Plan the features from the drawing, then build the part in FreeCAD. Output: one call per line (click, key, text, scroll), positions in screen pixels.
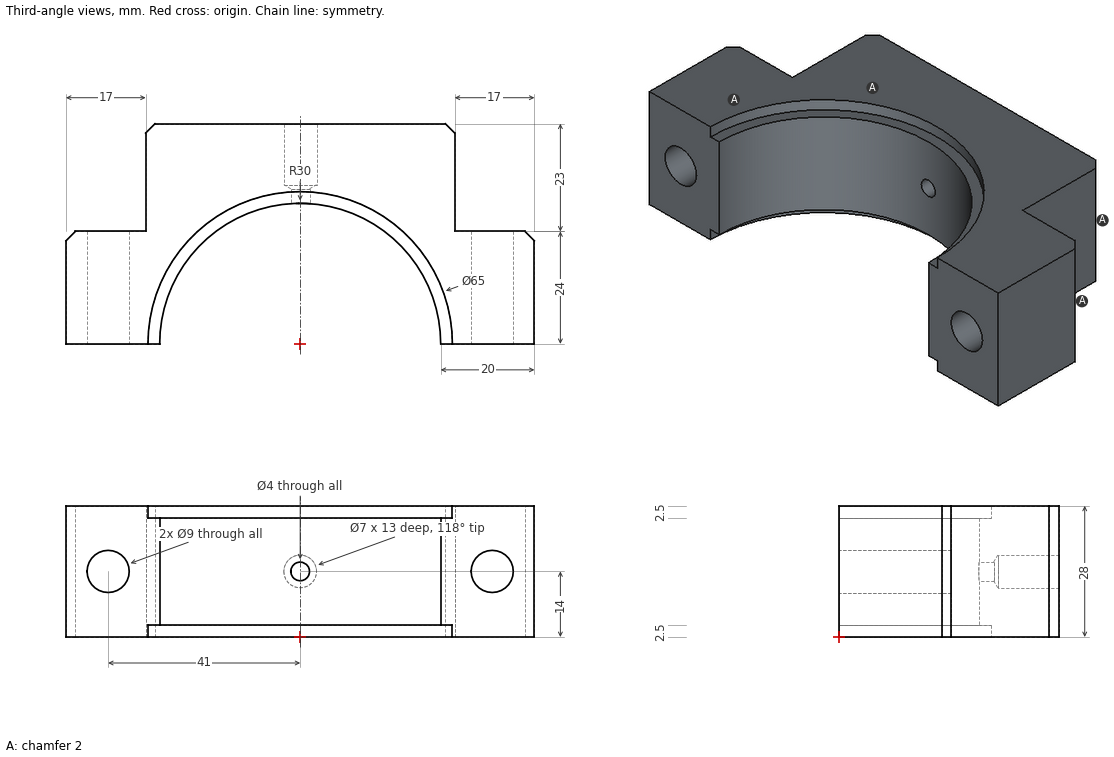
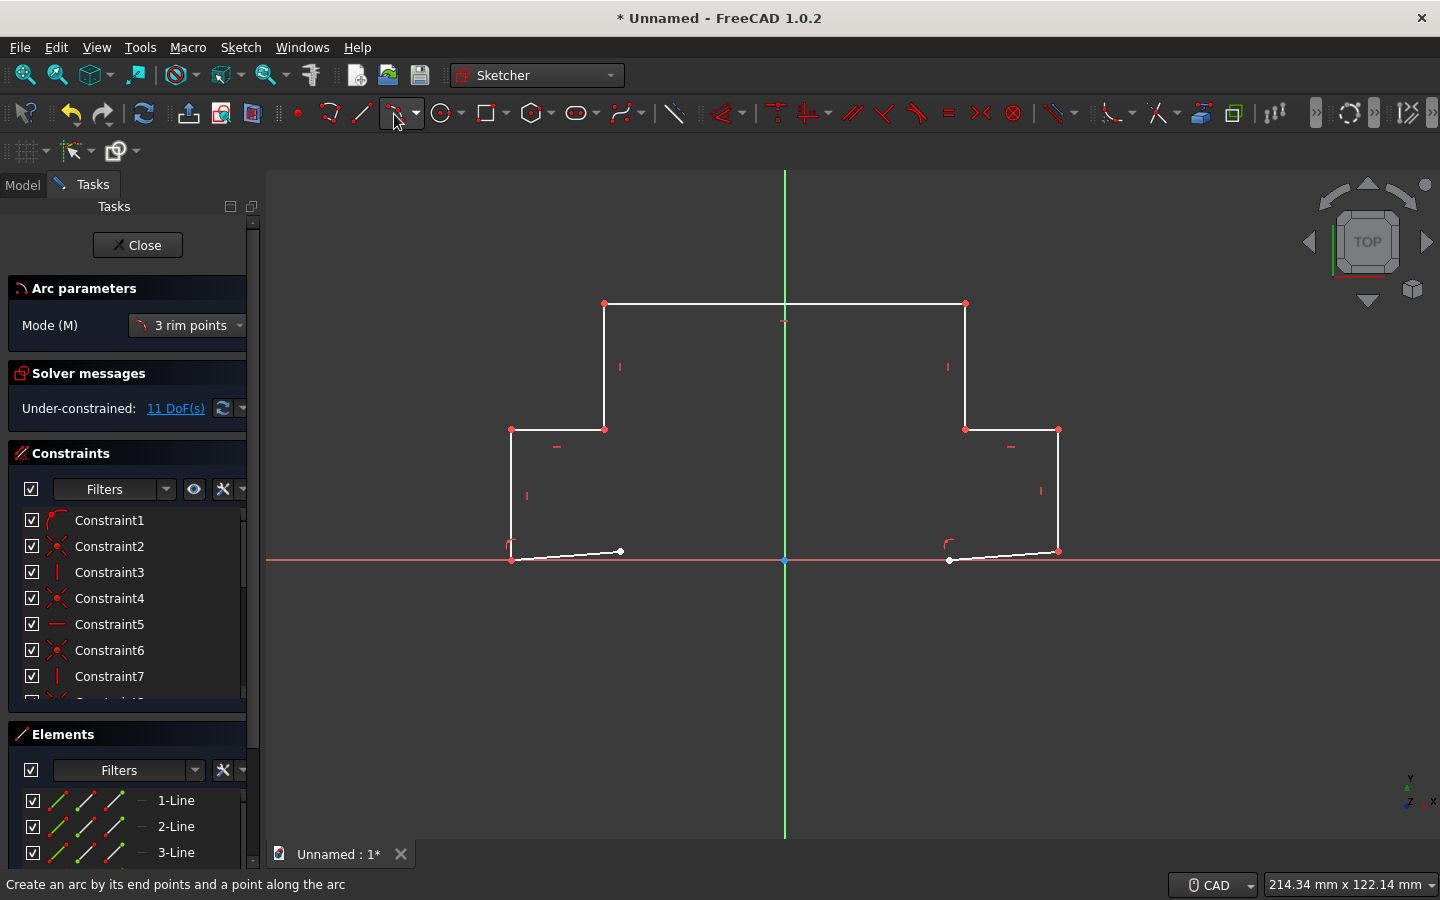
click(620, 552)
click(949, 560)
click(835, 404)
key(Escape)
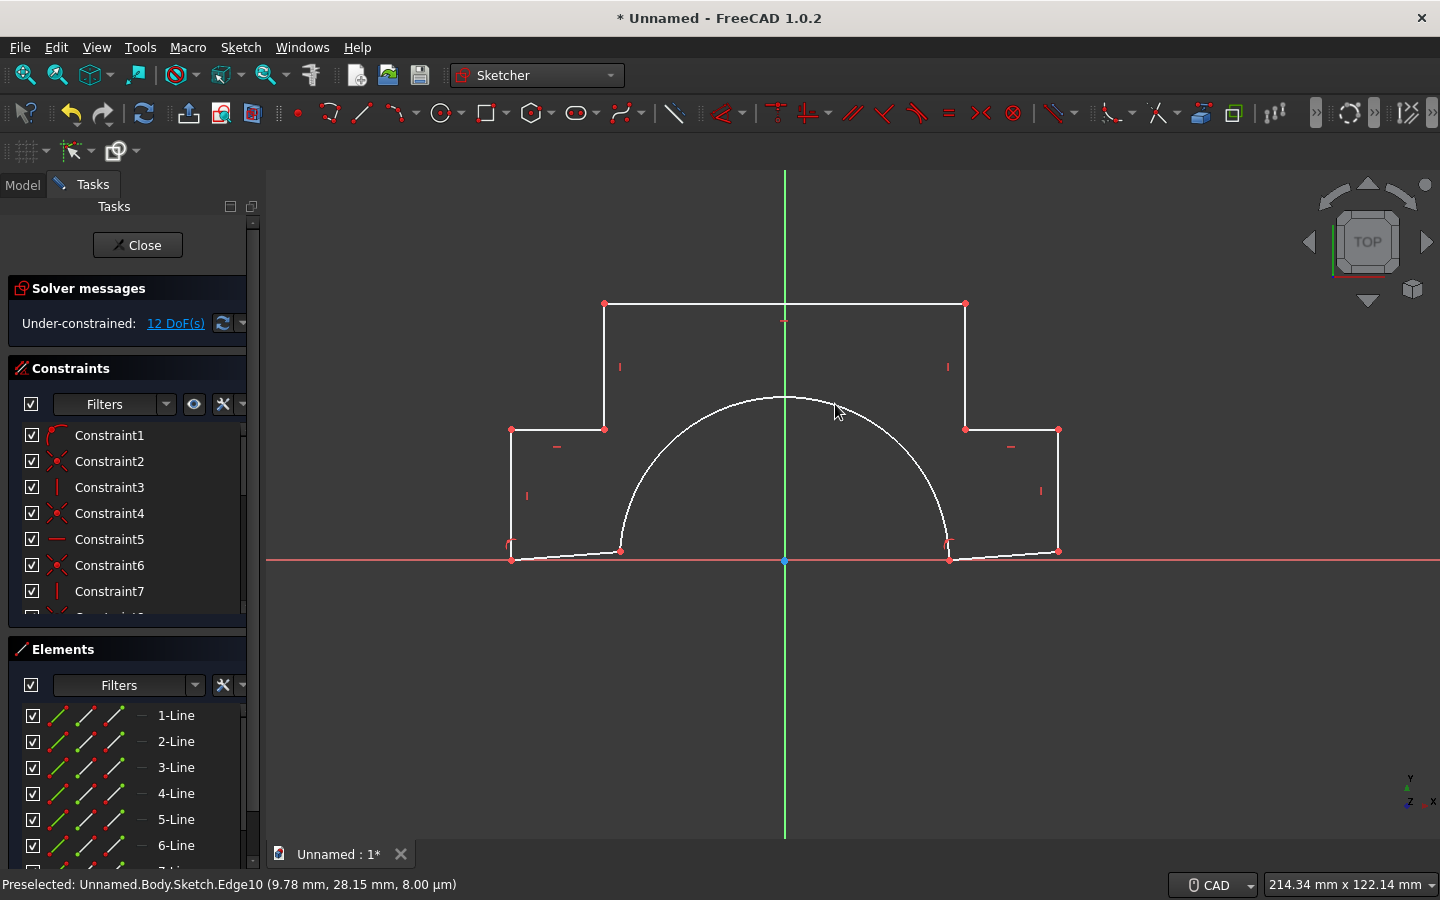
click(982, 558)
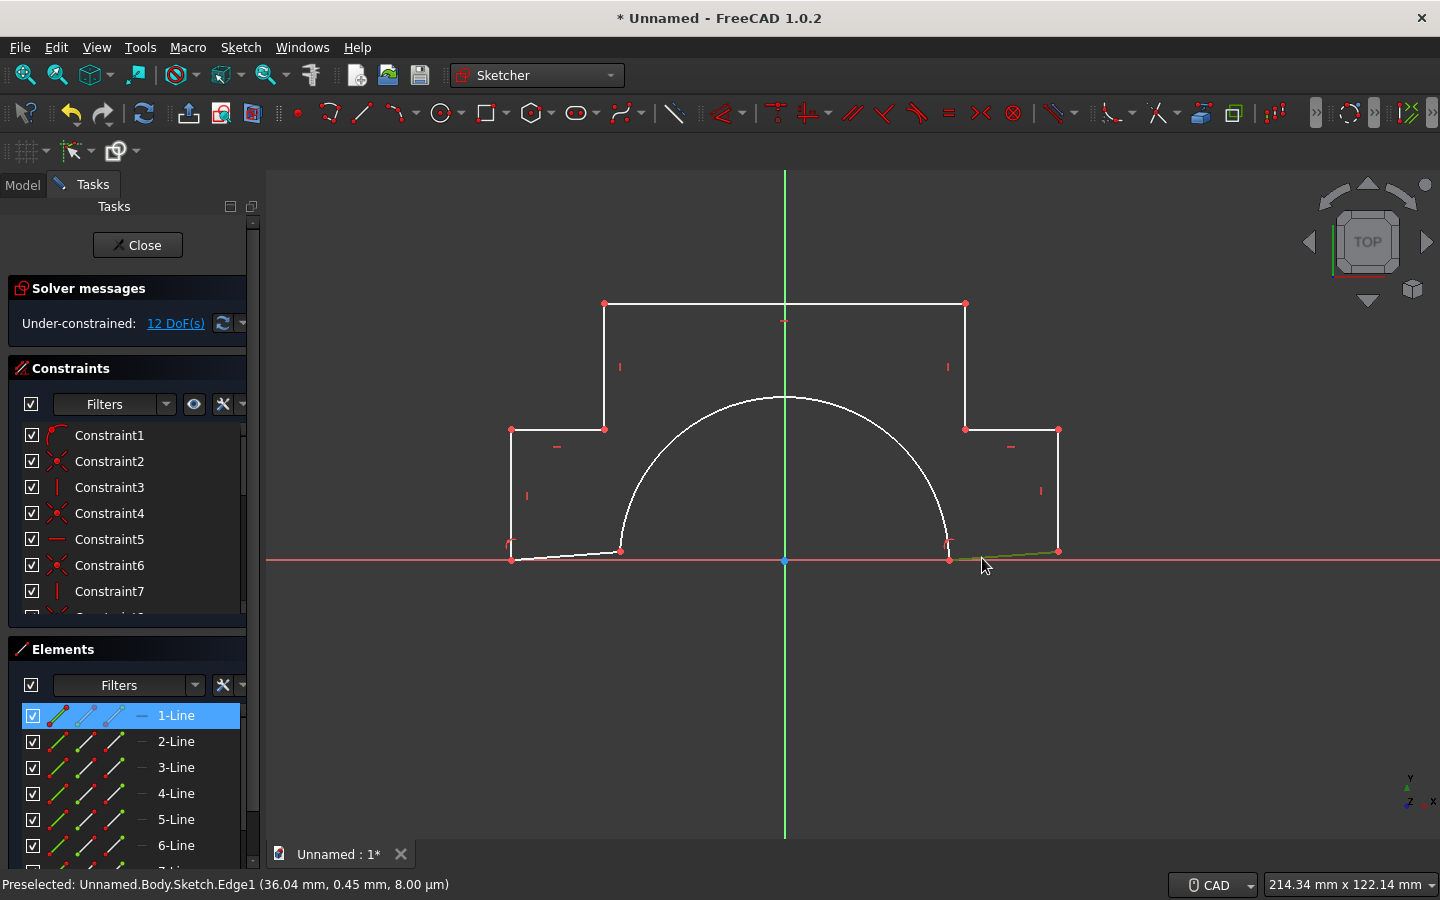
click(830, 114)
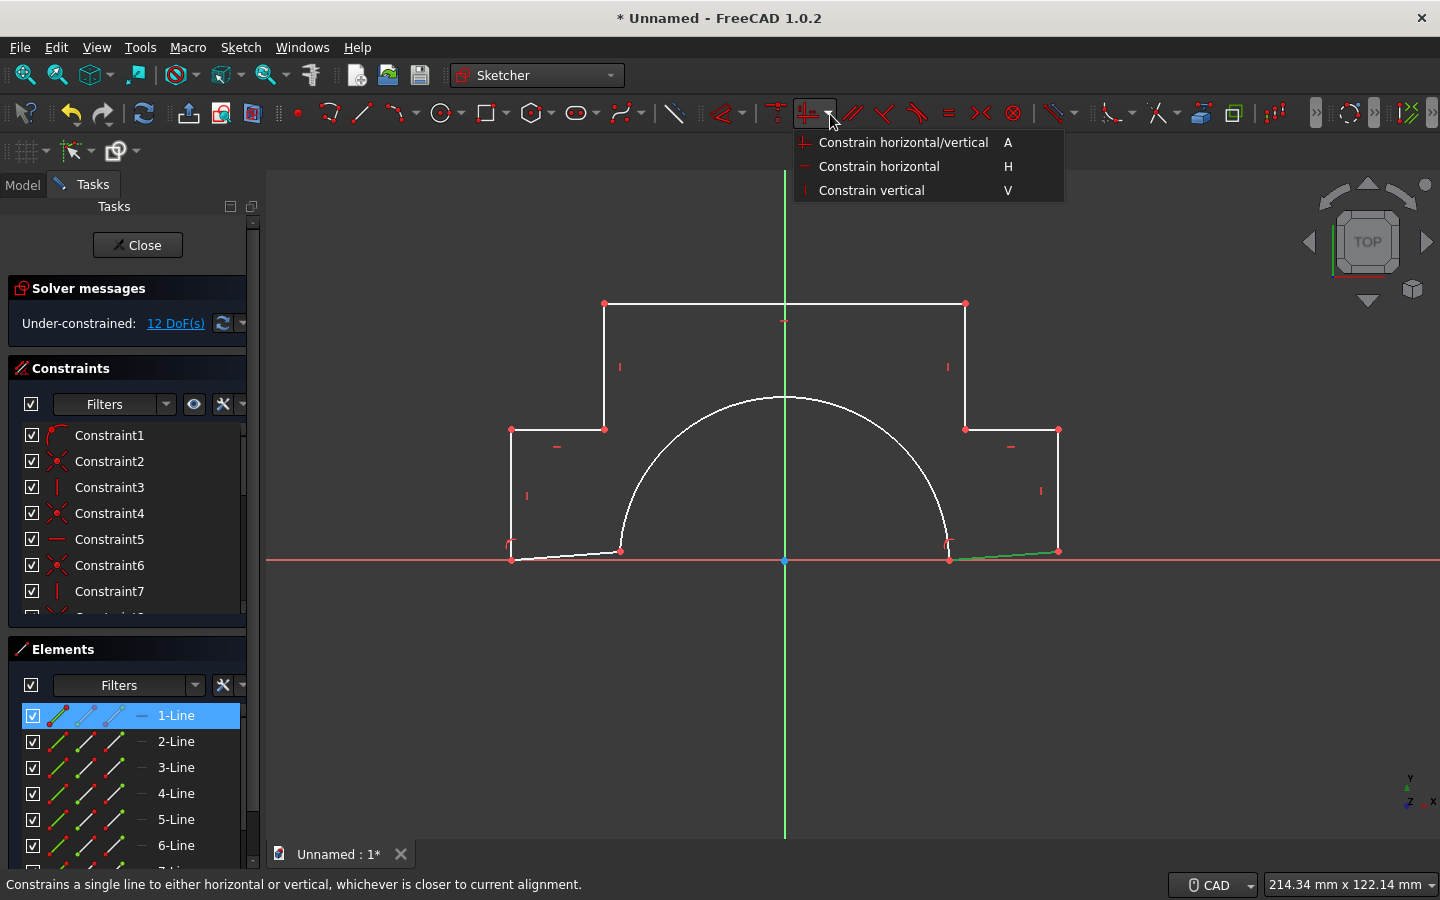
click(929, 166)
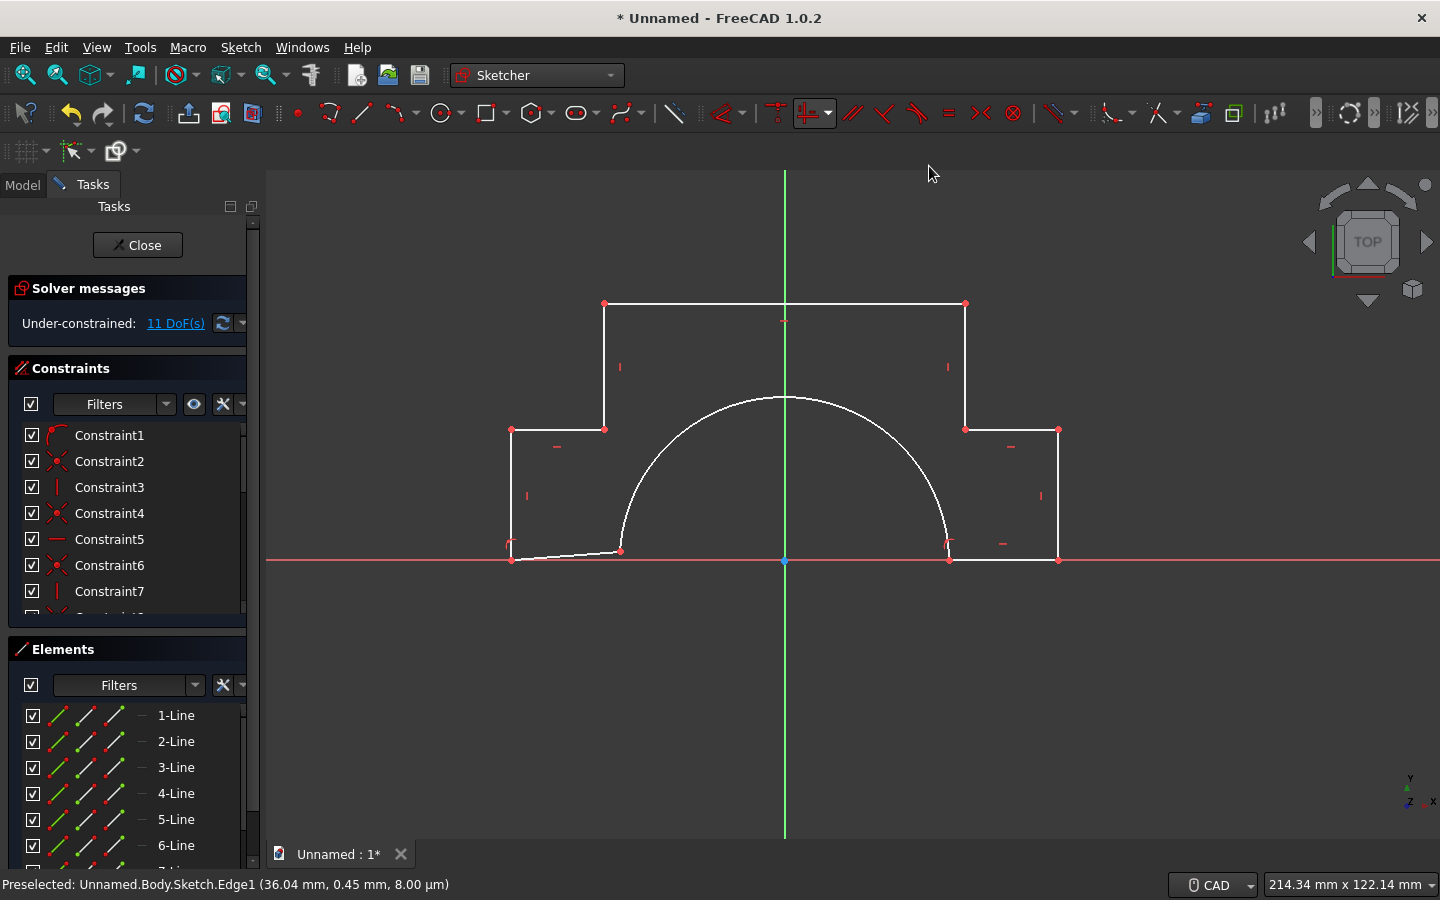
click(544, 558)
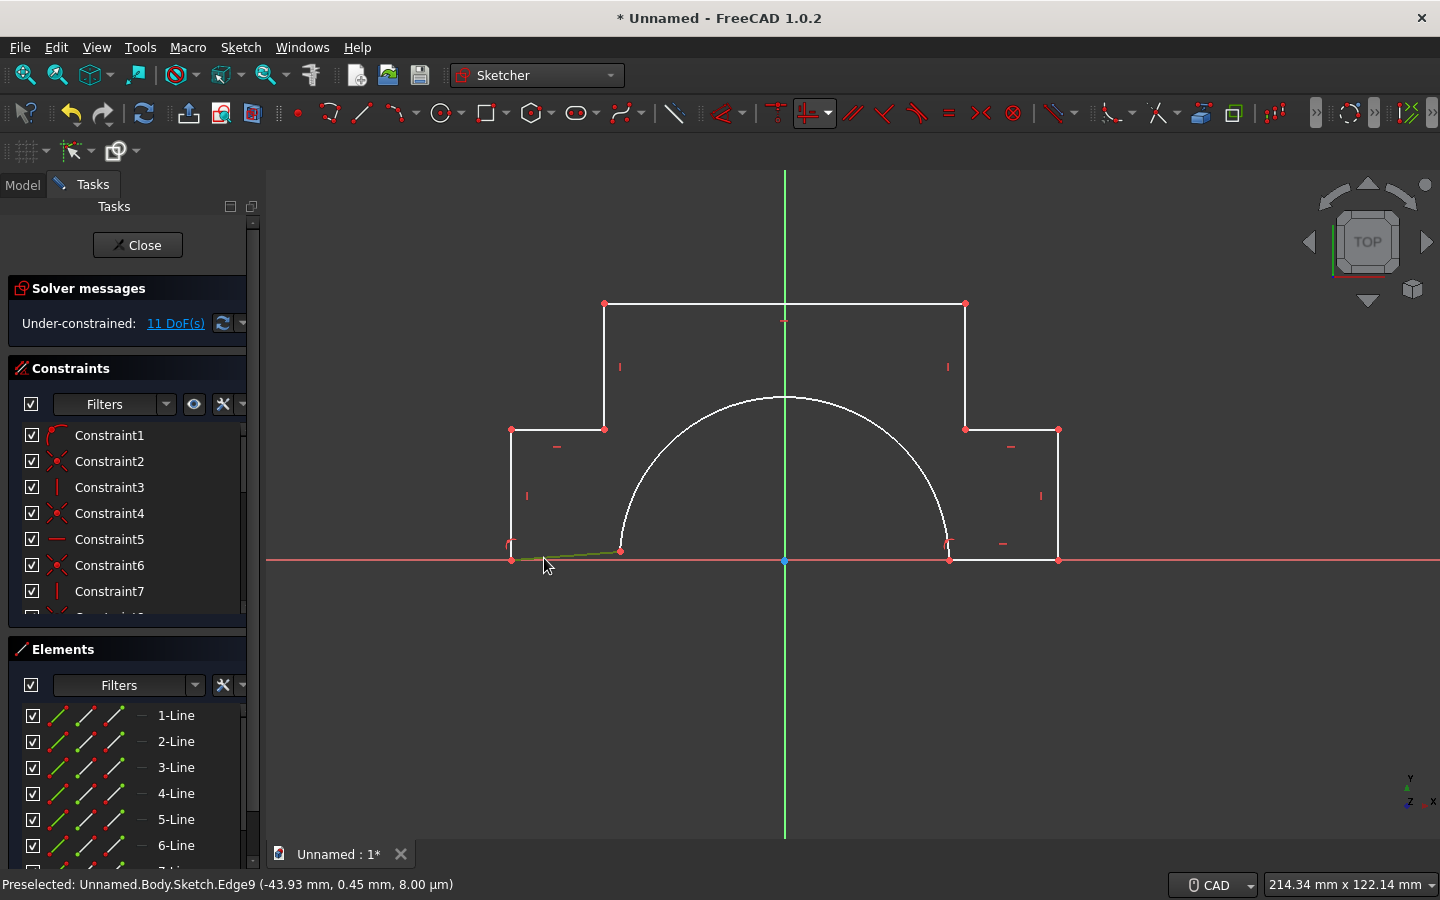
key(h)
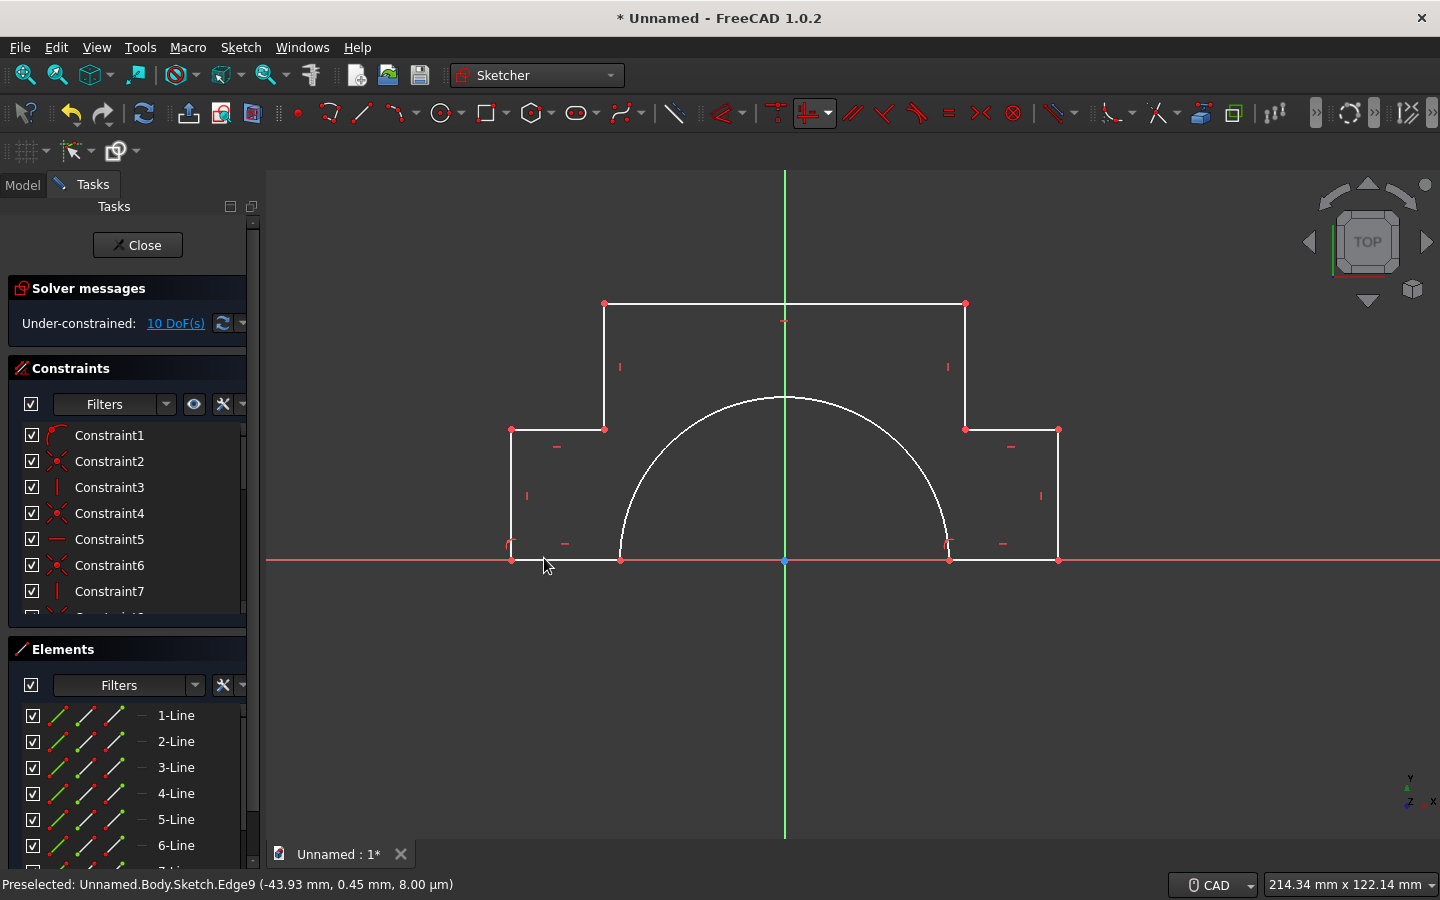
drag(774, 550, 795, 572)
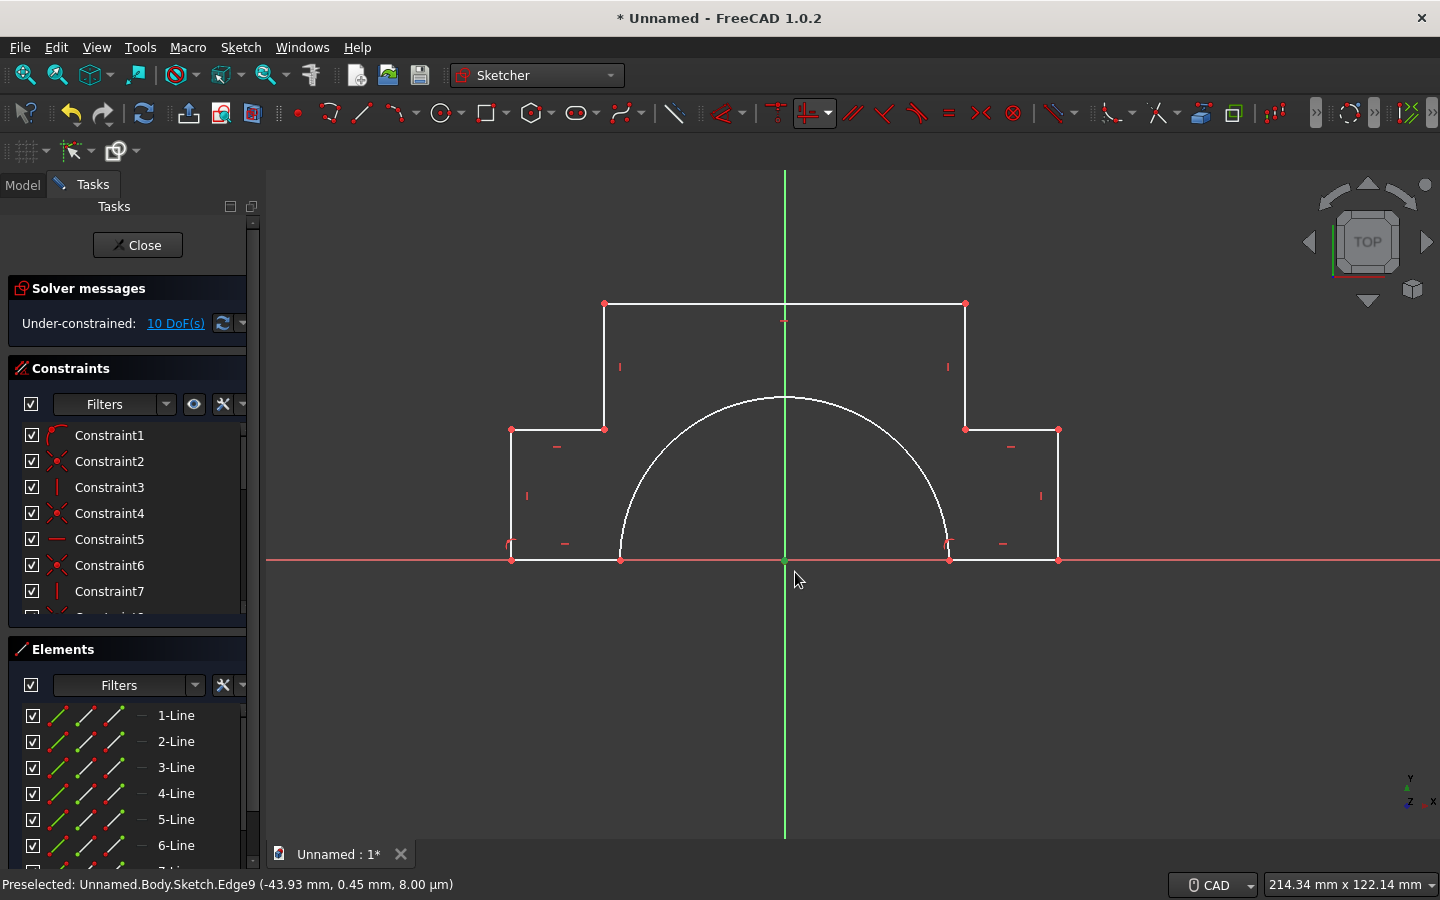
click(776, 114)